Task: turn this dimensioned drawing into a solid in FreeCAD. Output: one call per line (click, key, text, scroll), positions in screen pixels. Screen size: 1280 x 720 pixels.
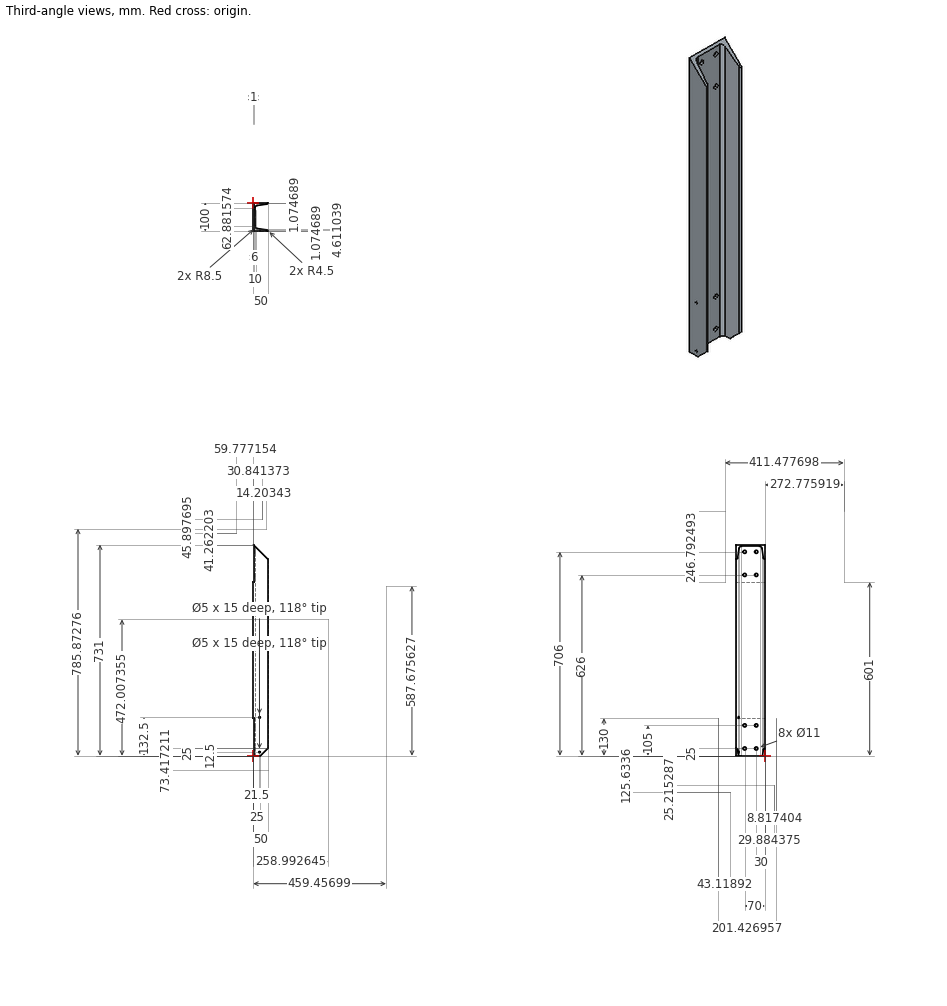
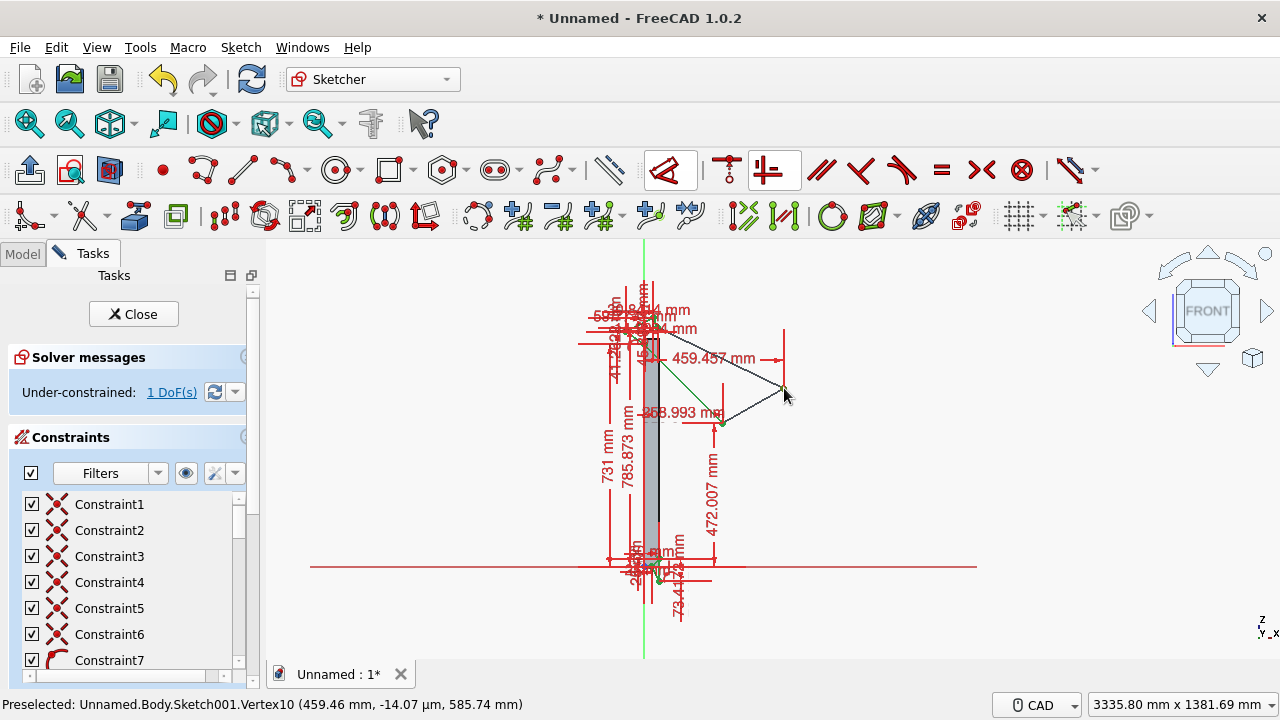
key(i)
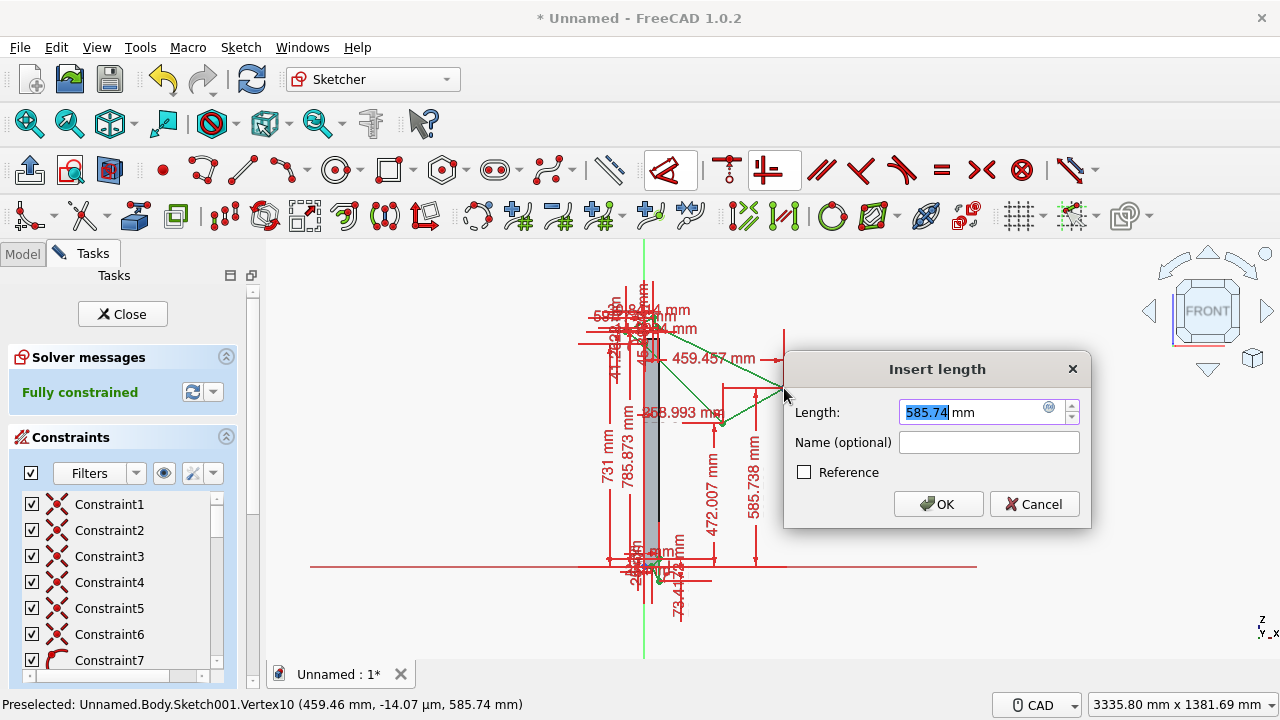
text(587.675627)
key(Return)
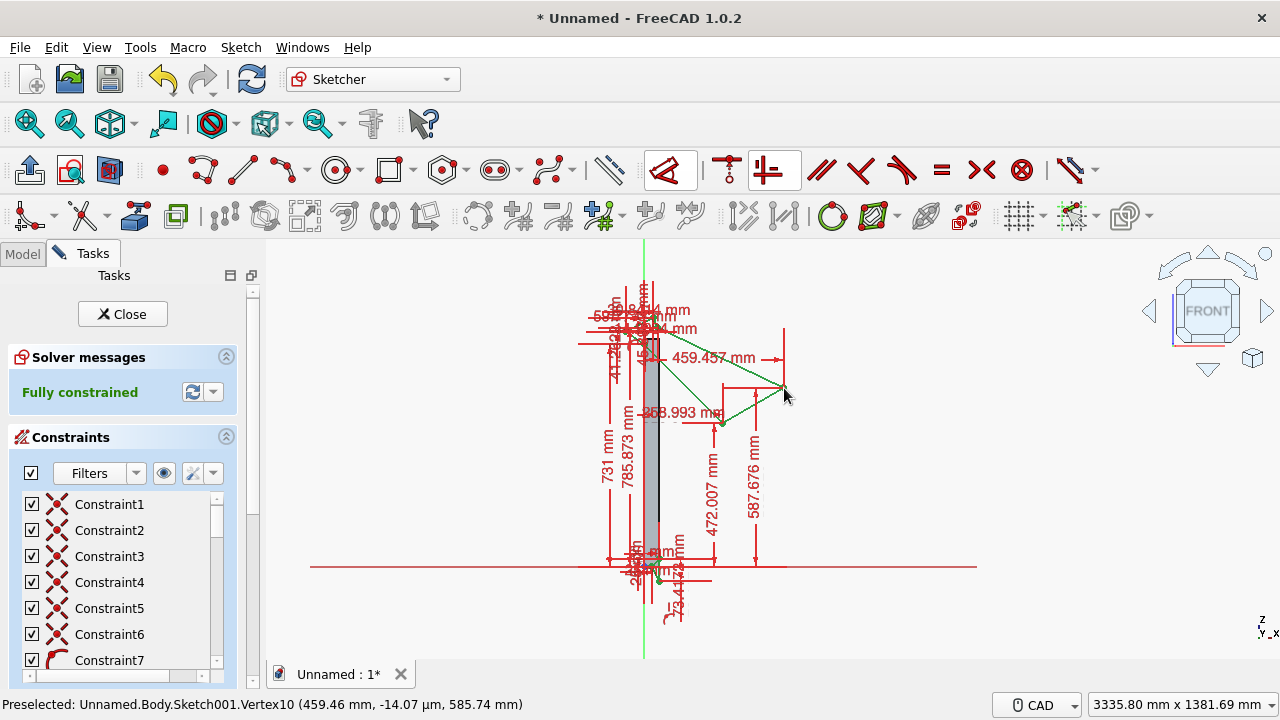
click(123, 314)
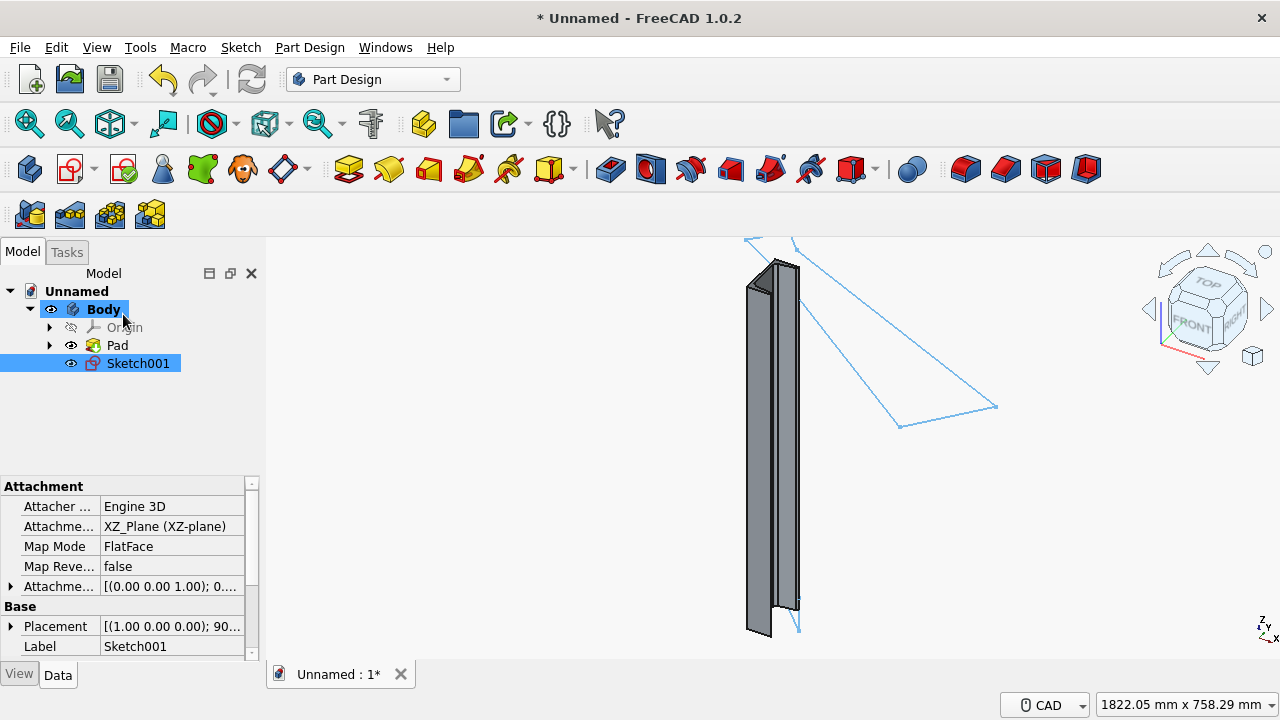
click(612, 170)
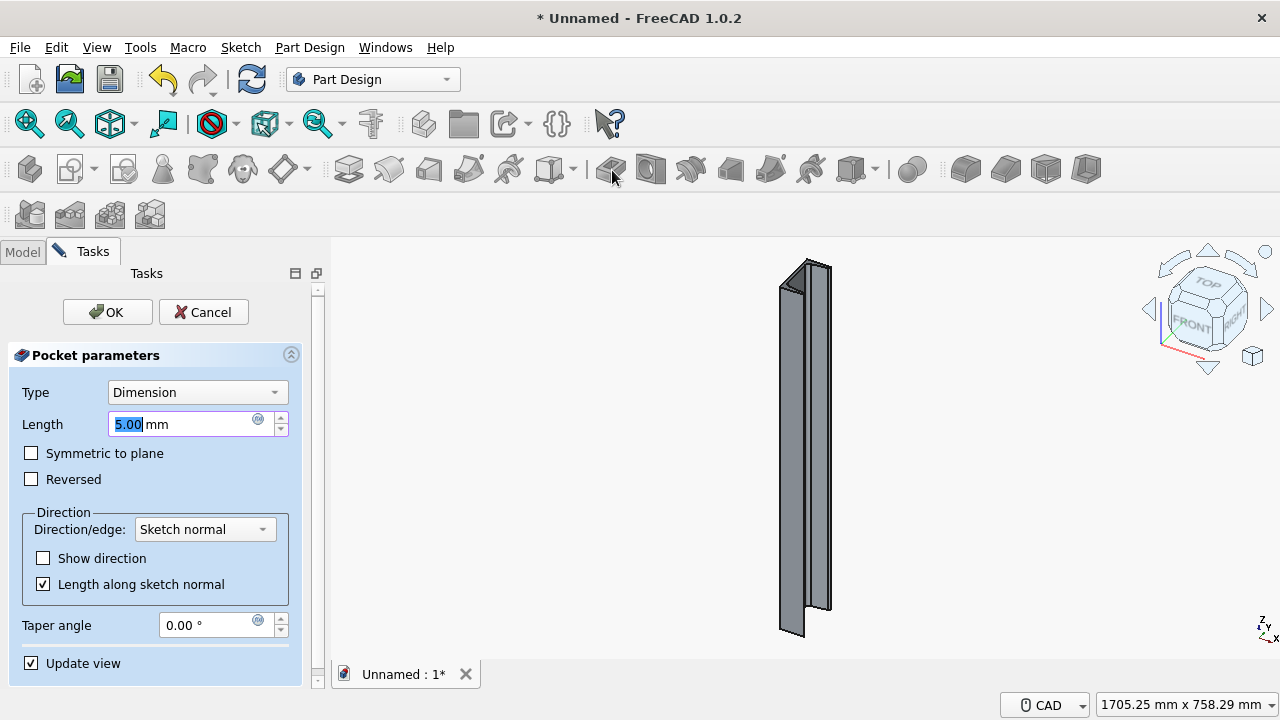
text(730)
key(Tab)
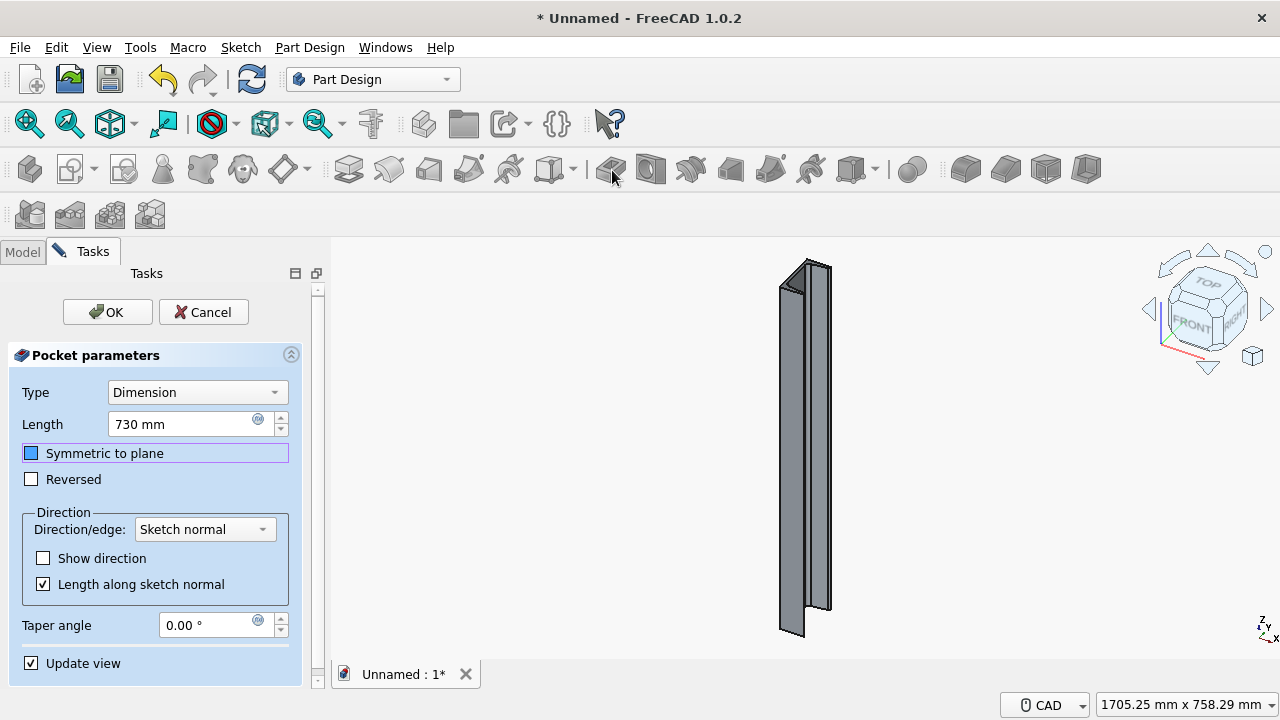
click(30, 479)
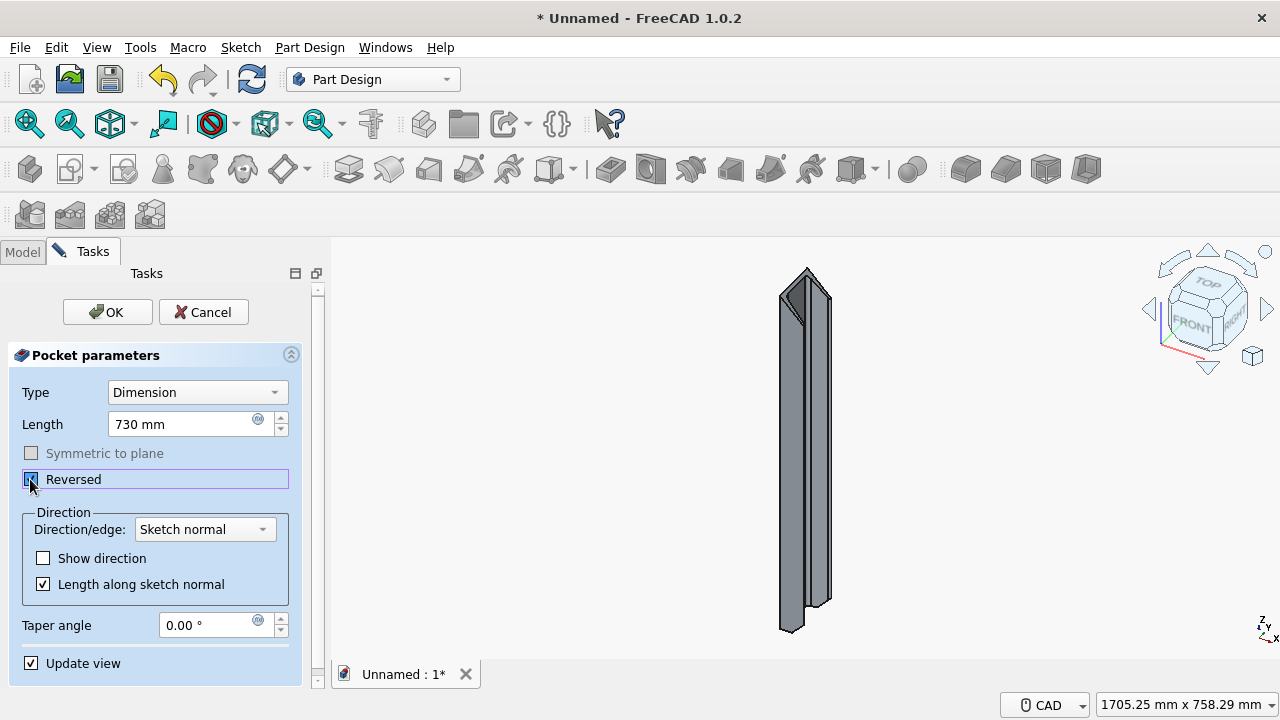
click(108, 312)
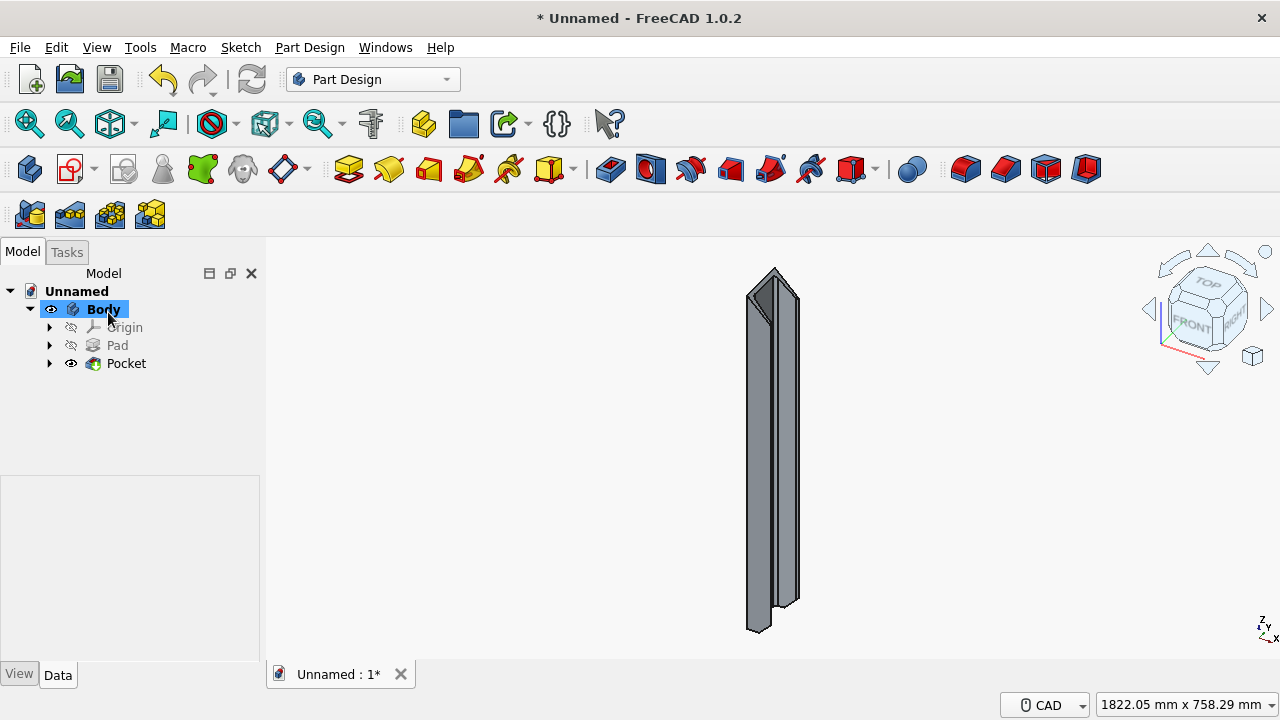
key(6)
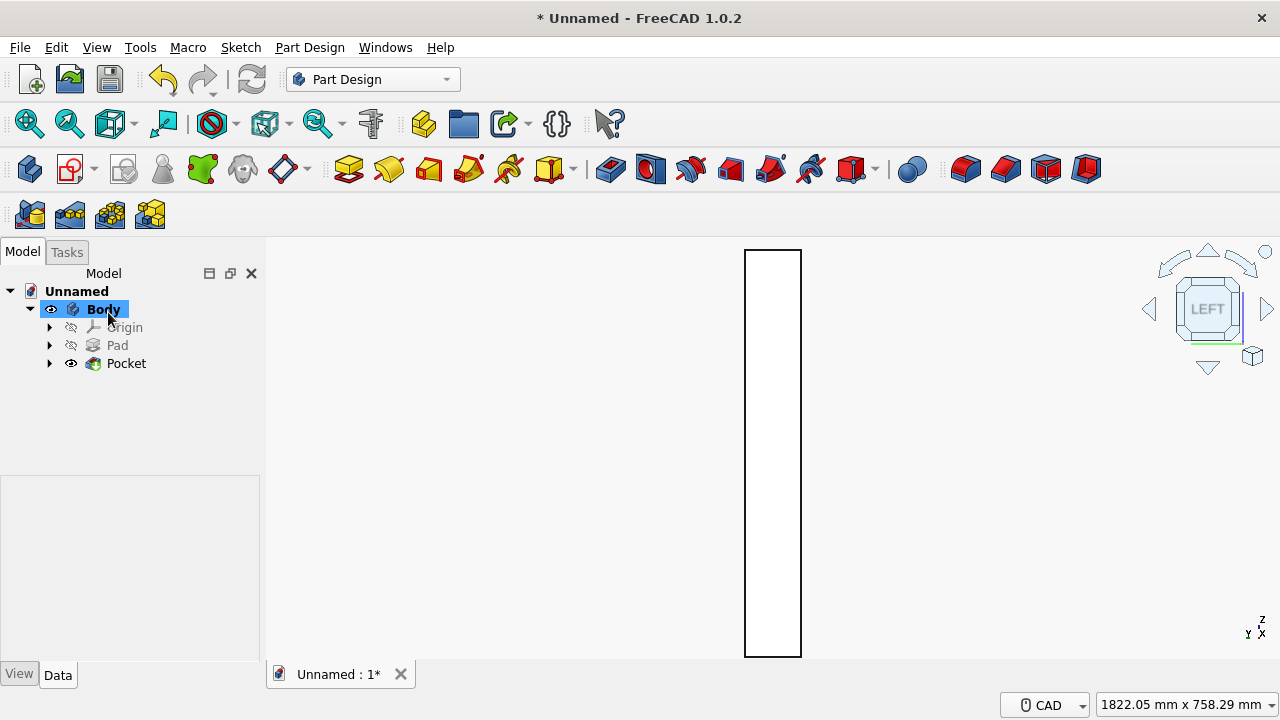
click(773, 278)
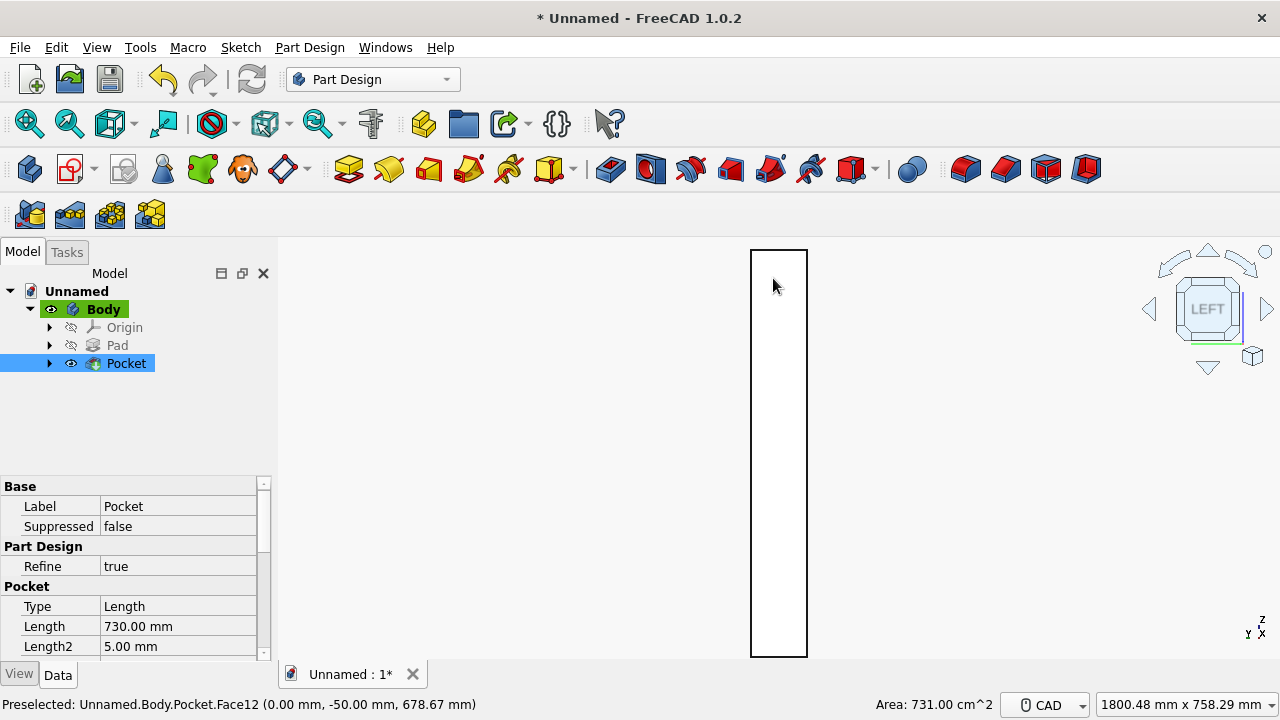
click(70, 170)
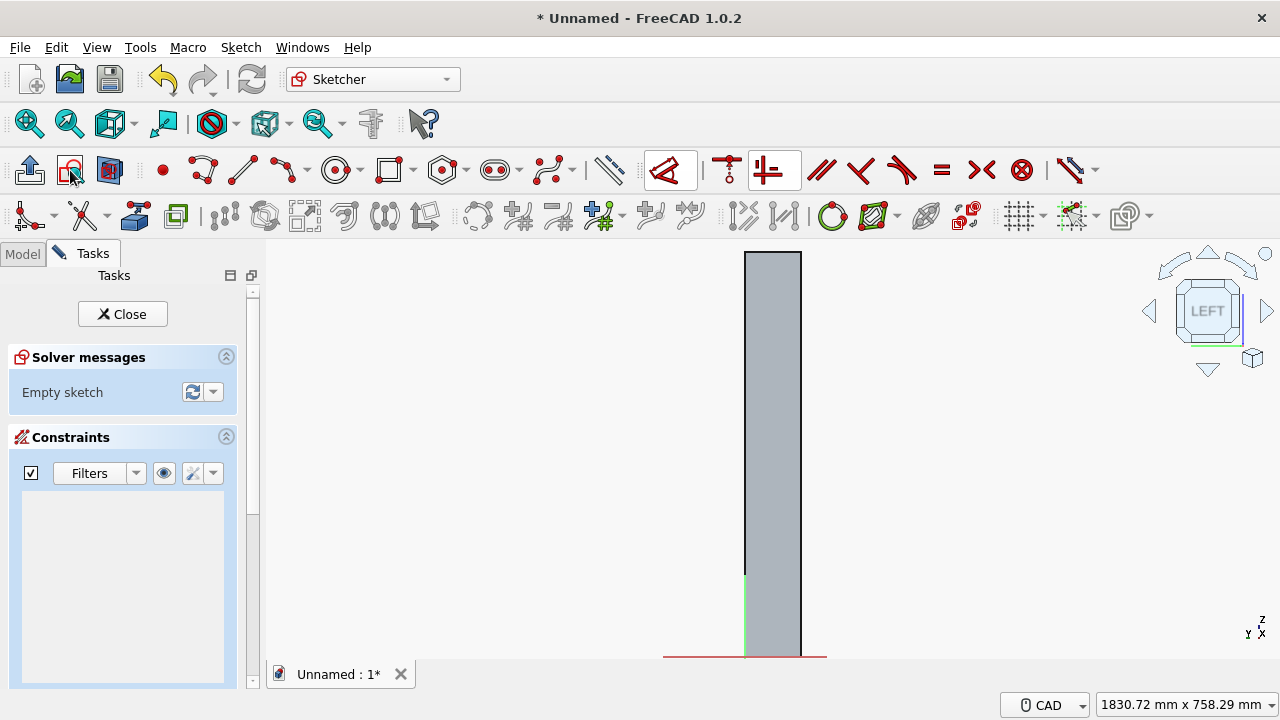
scroll(696, 443, down, 4)